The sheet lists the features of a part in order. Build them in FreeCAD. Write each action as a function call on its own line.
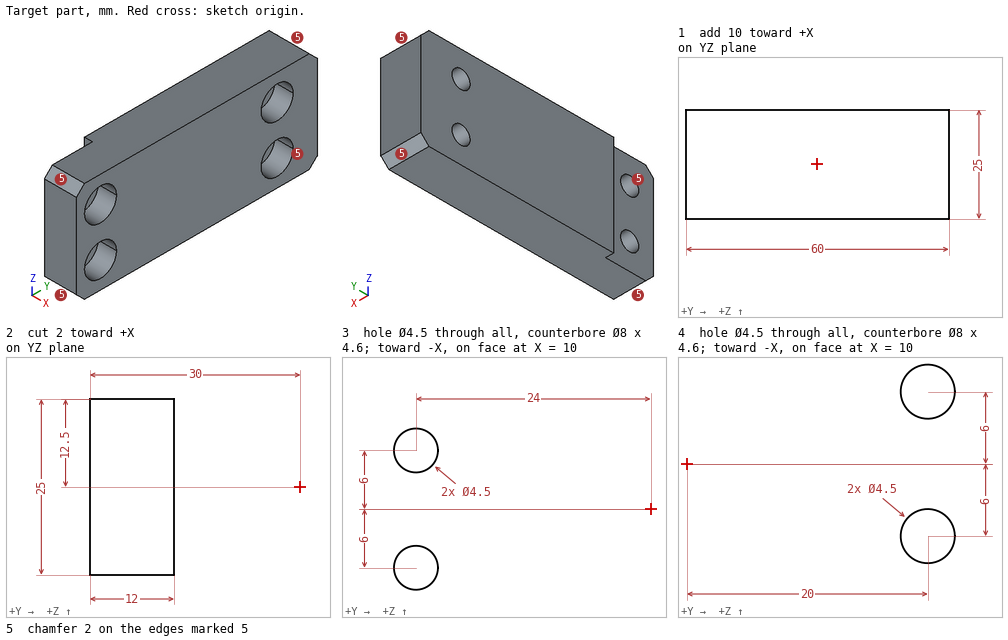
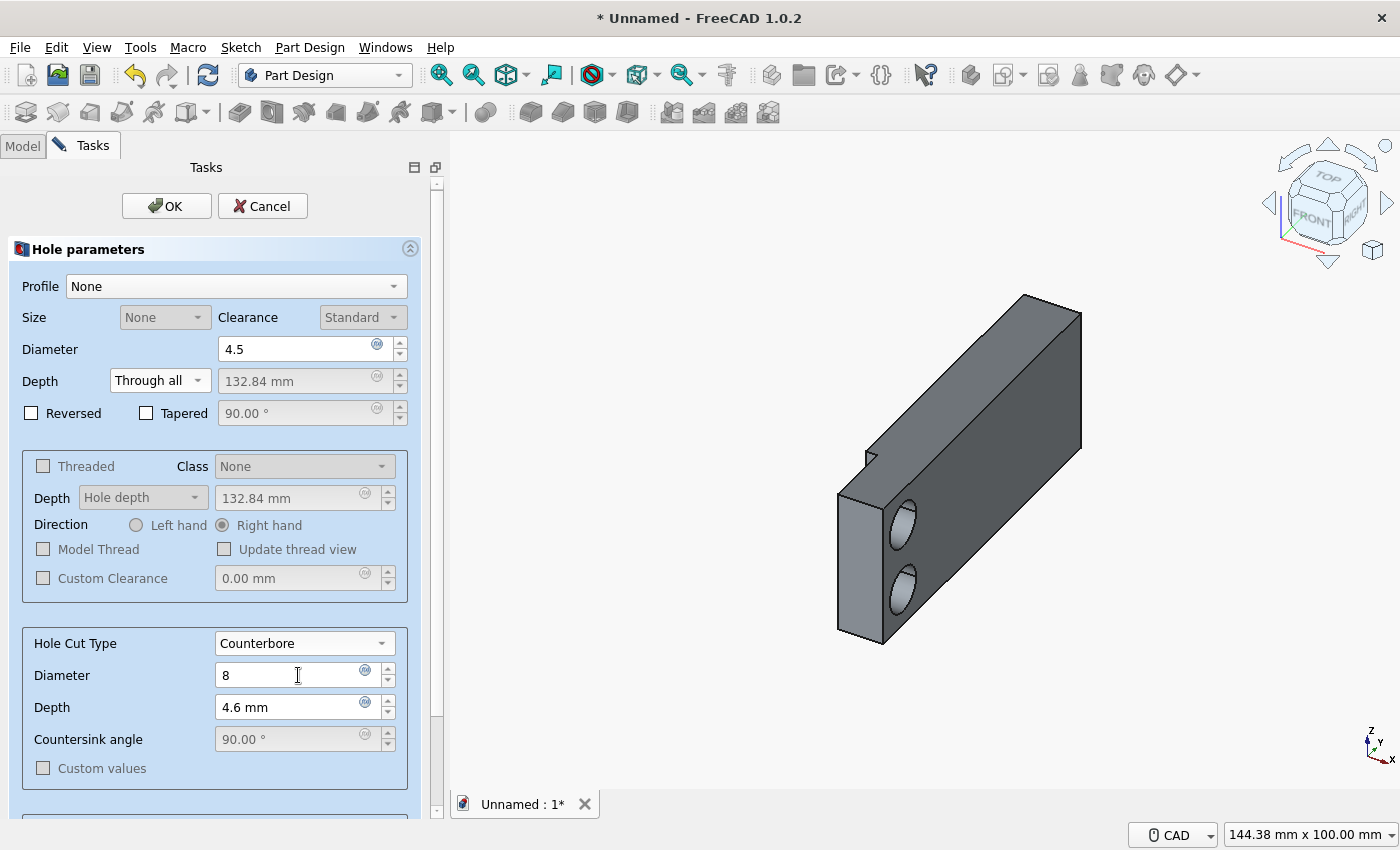
click(167, 206)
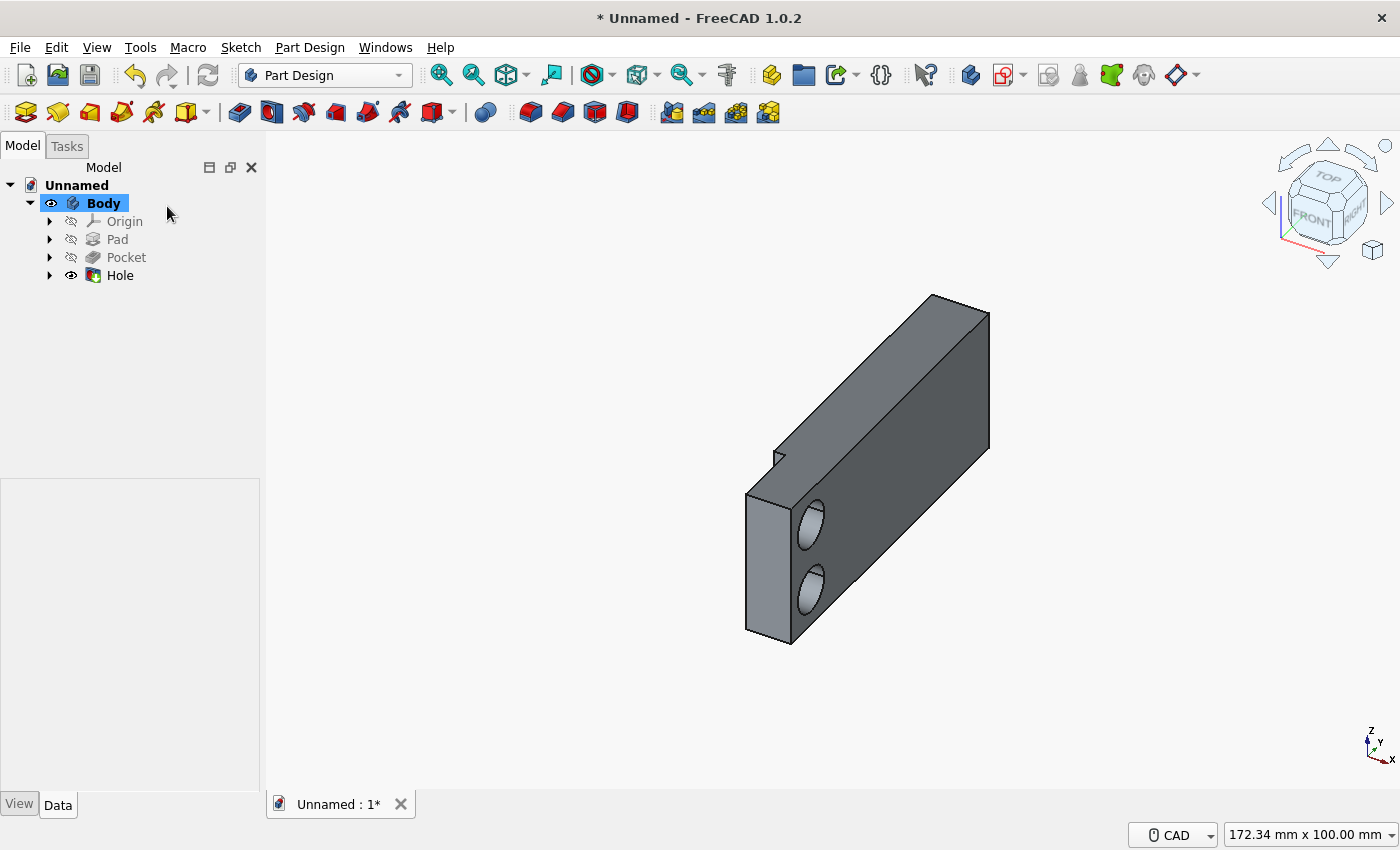
click(946, 422)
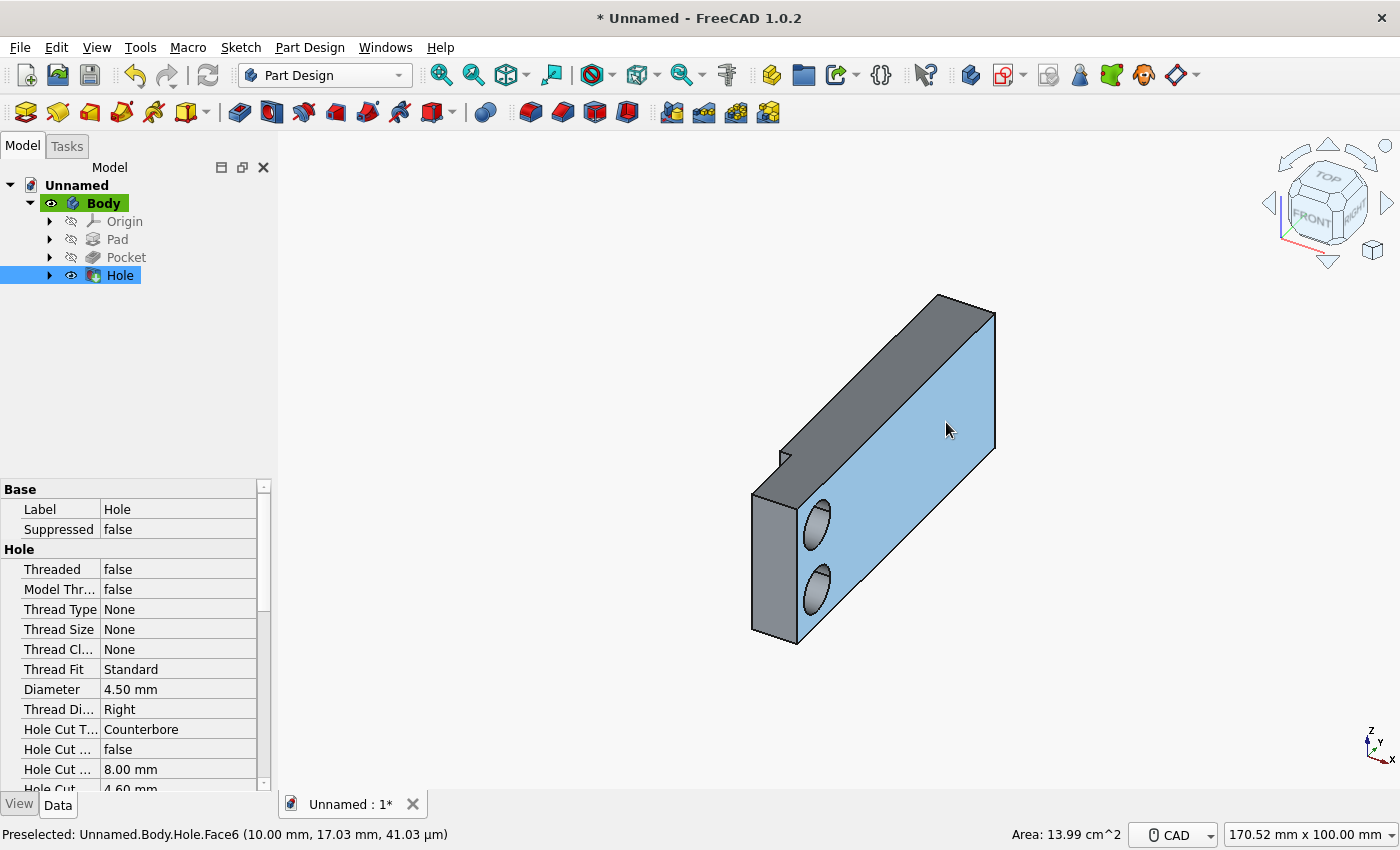
click(1004, 76)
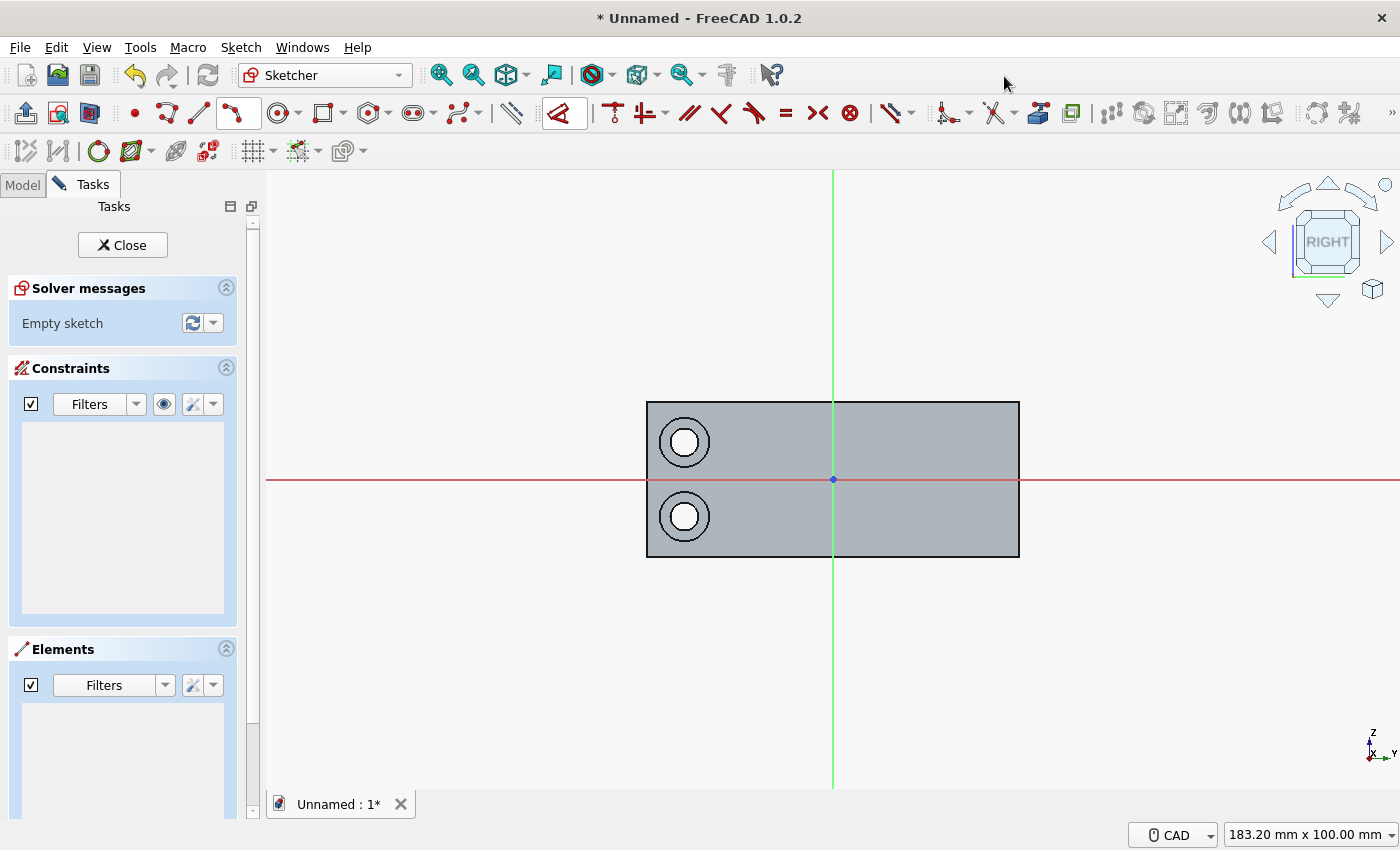
scroll(947, 480, up, 7)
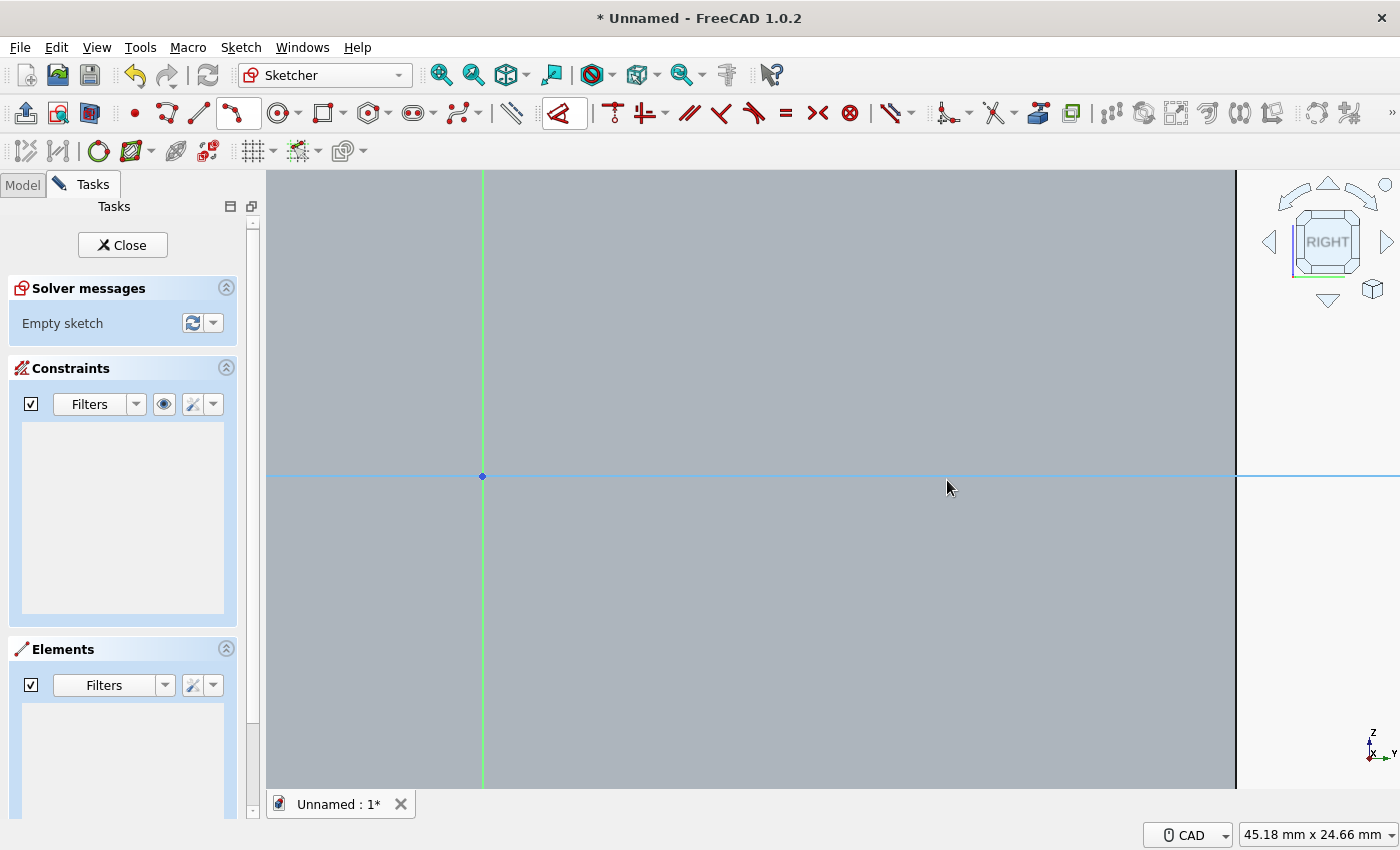
click(278, 114)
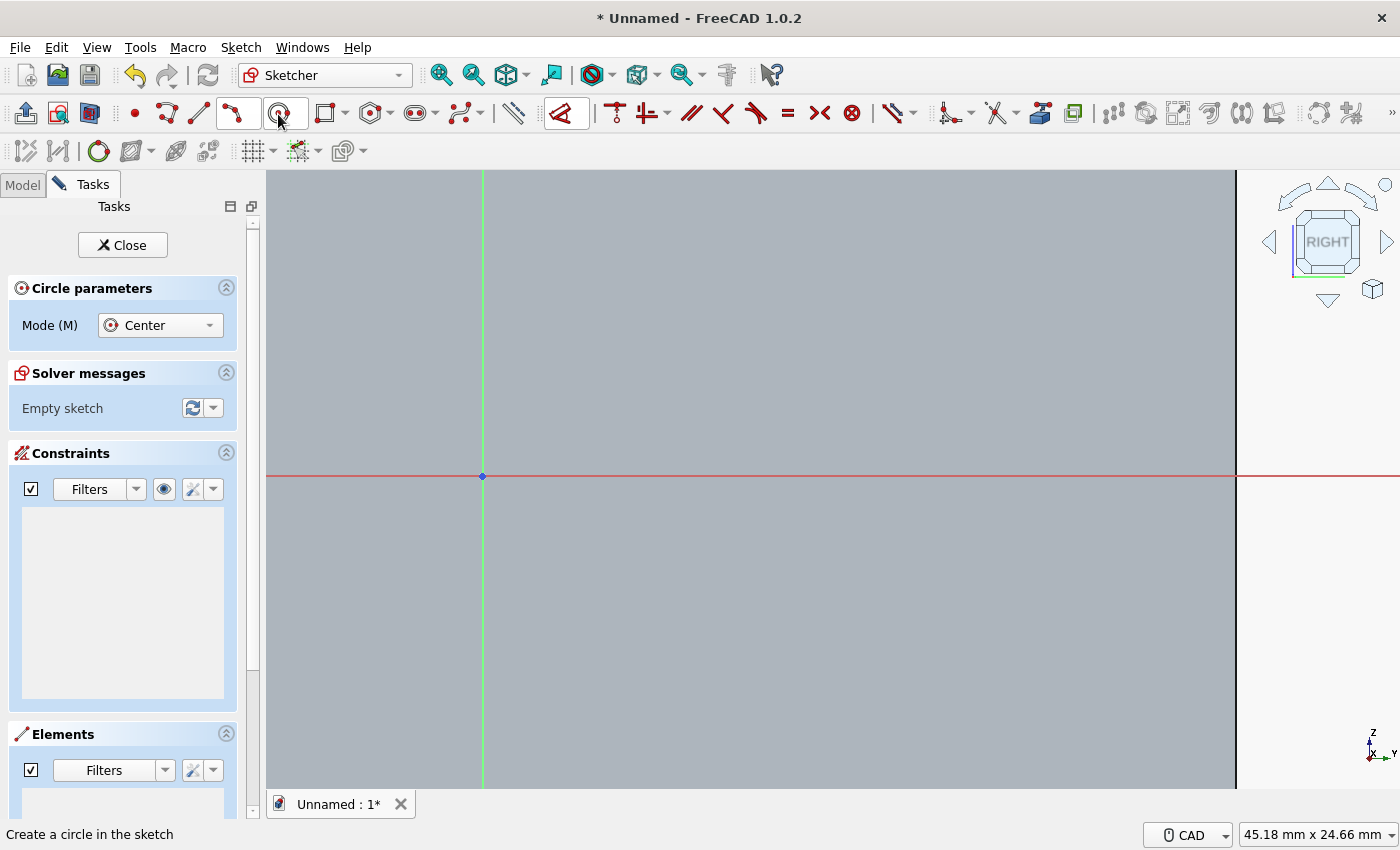
click(985, 627)
click(1025, 587)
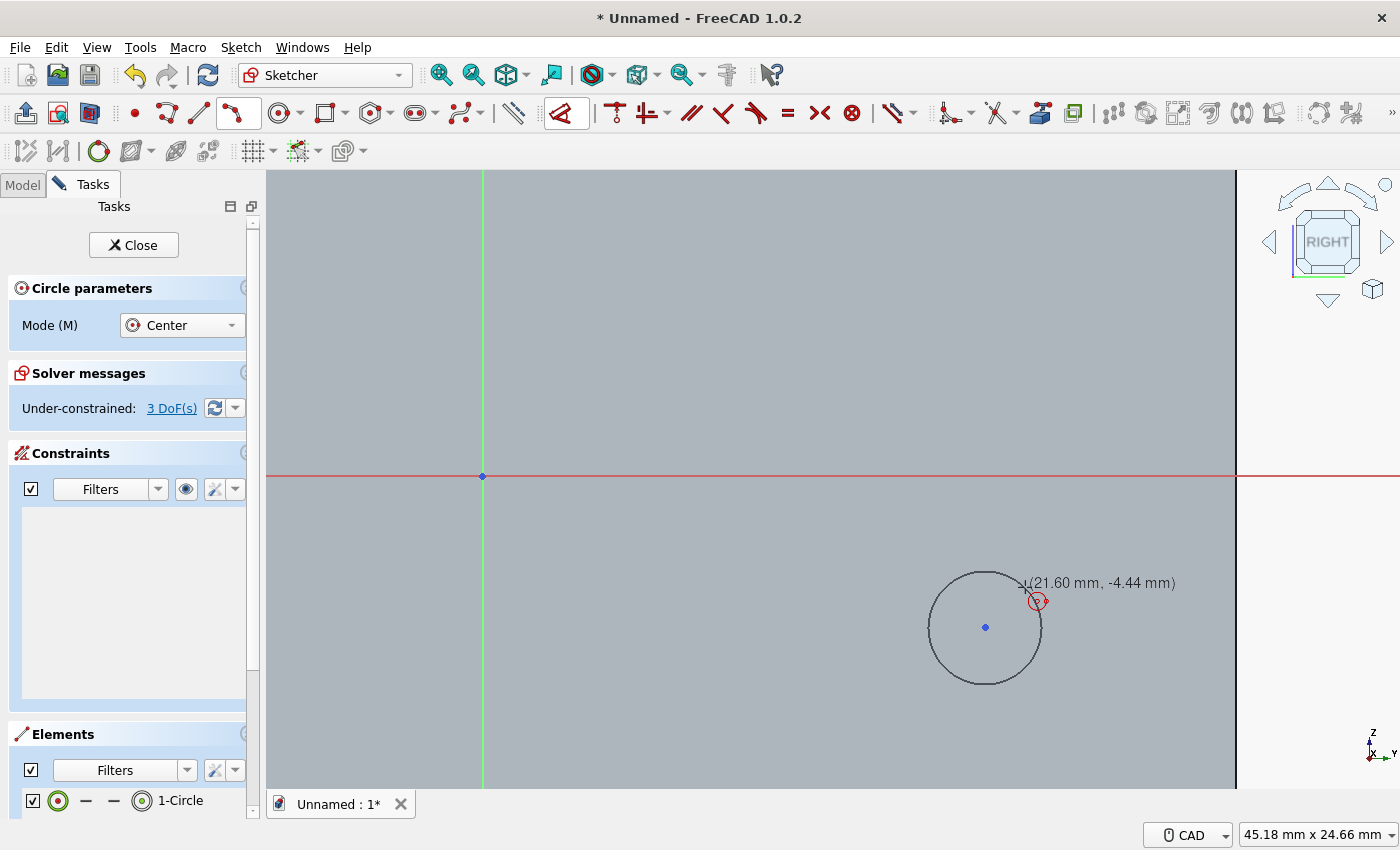
click(985, 326)
click(1025, 286)
key(Escape)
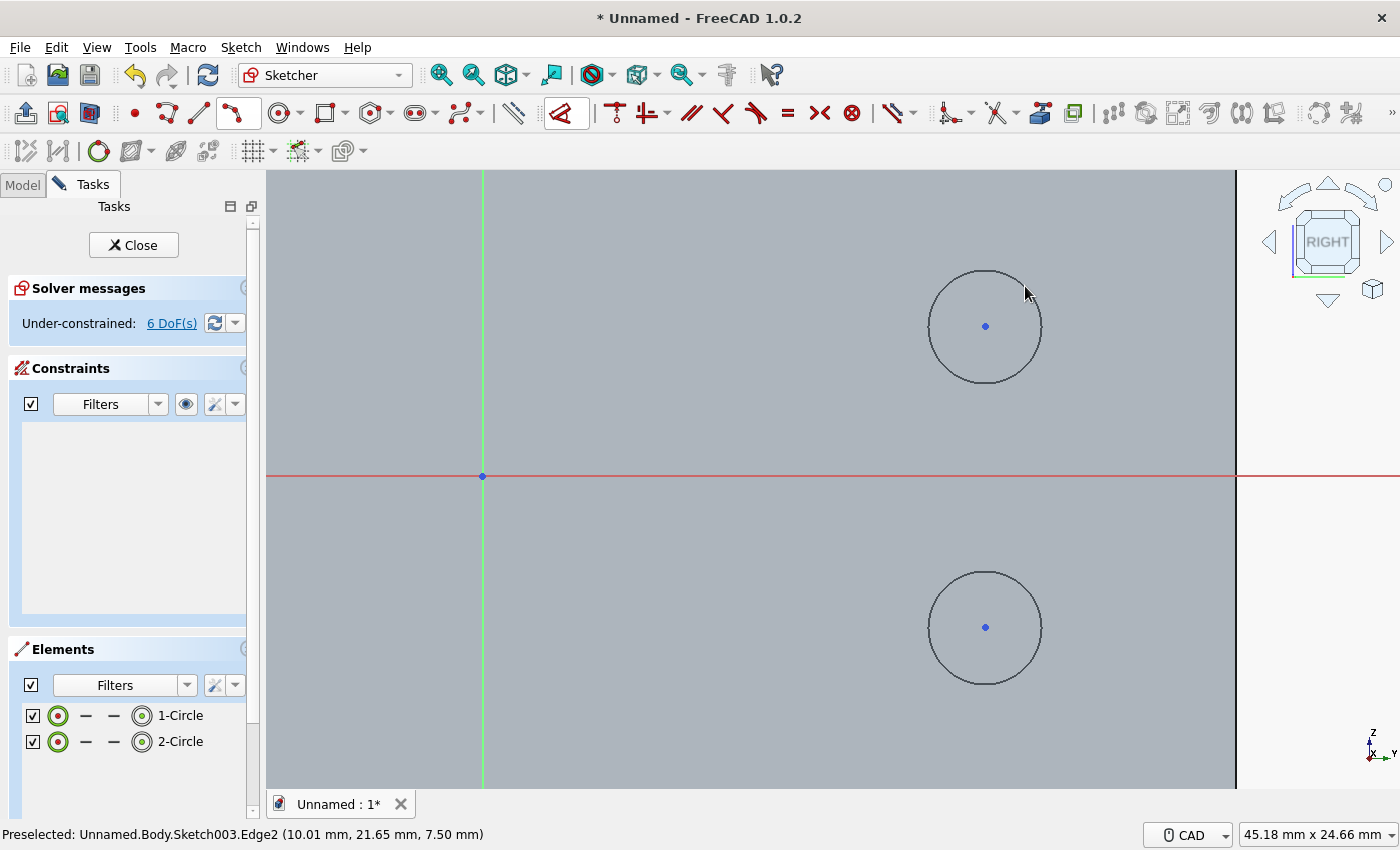
click(1025, 588)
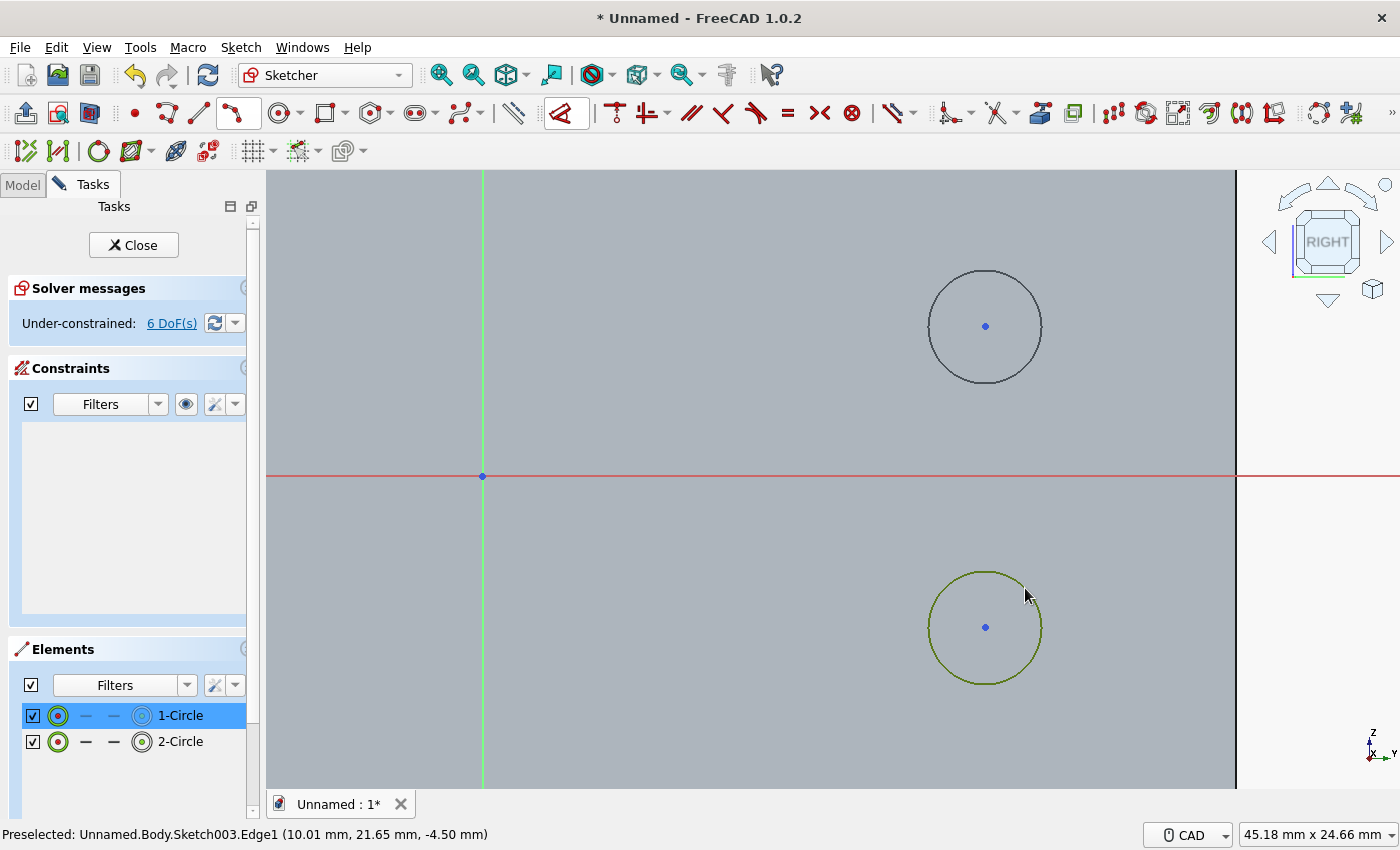
click(1025, 287)